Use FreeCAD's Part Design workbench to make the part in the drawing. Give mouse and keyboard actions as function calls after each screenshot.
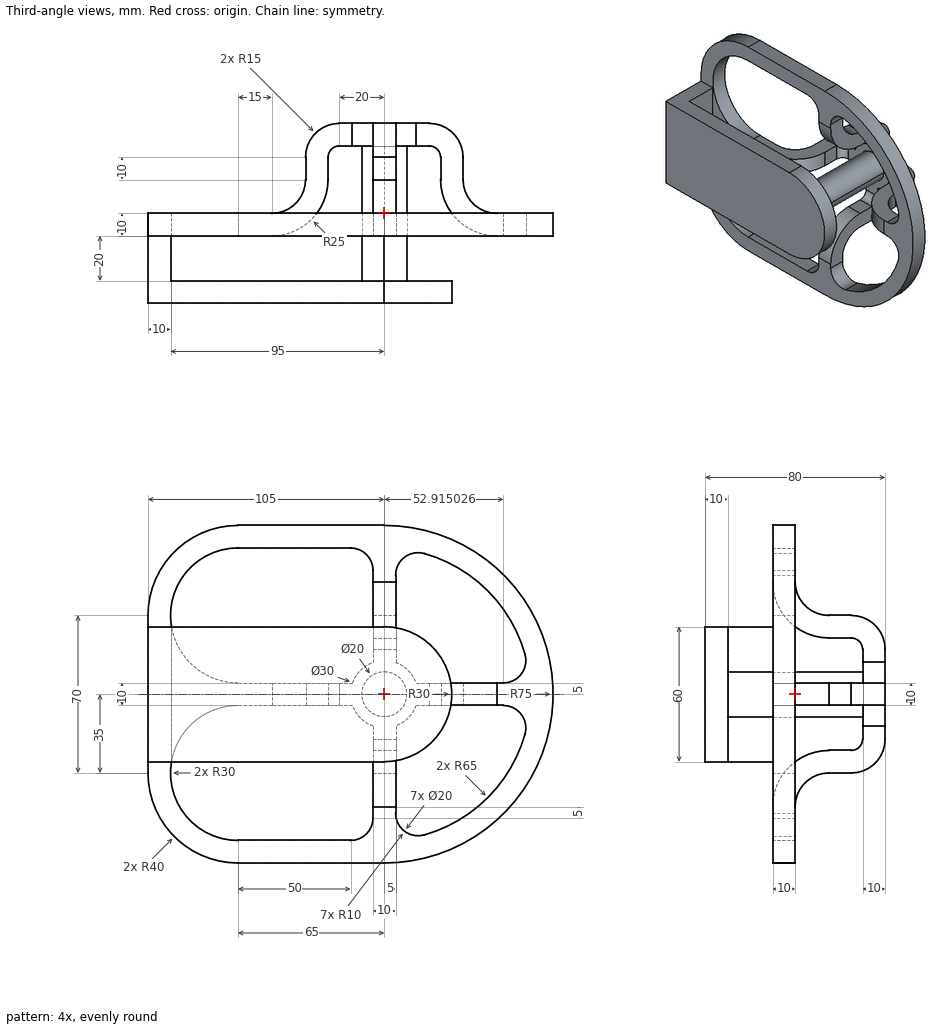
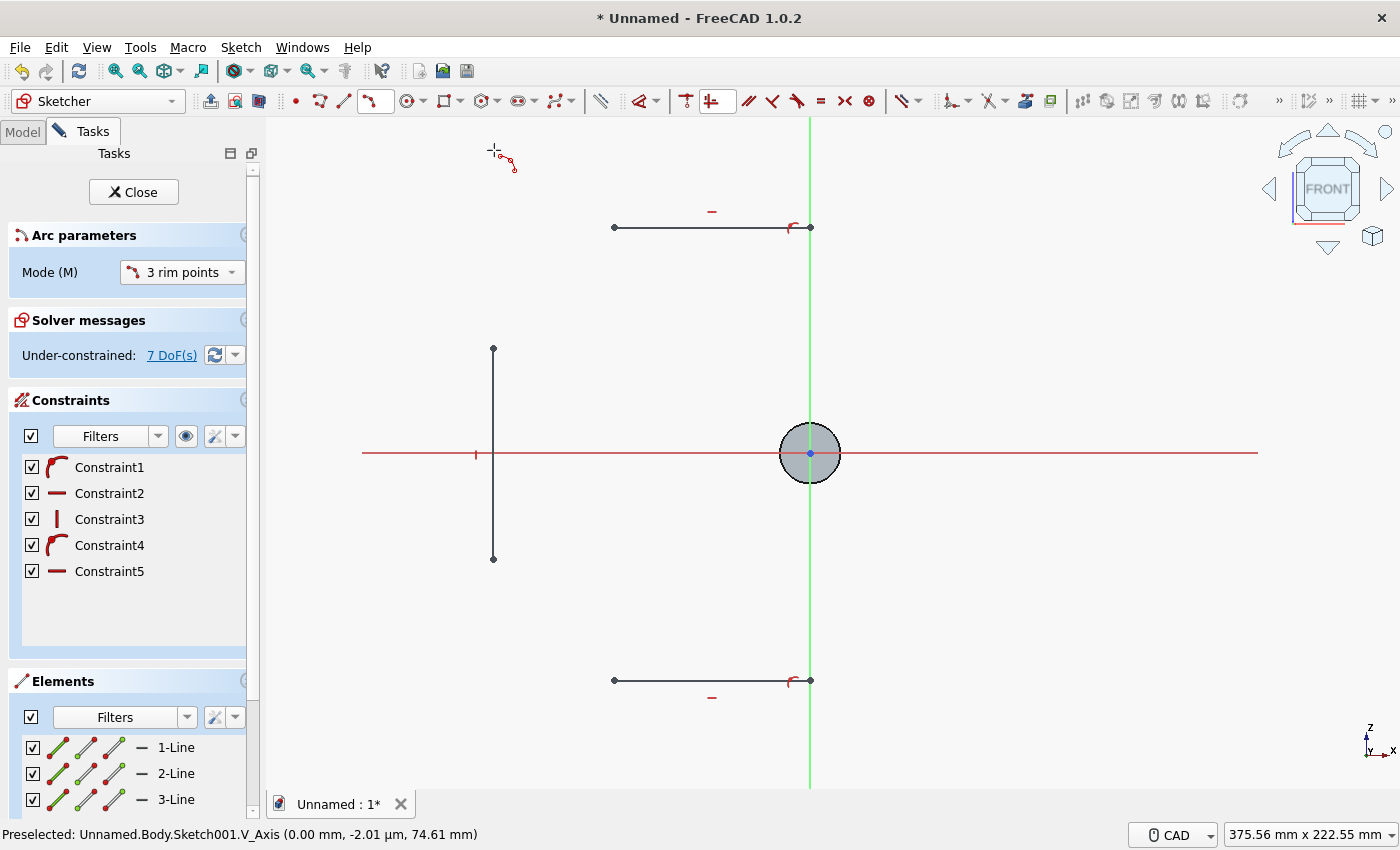
click(614, 681)
click(493, 560)
click(528, 644)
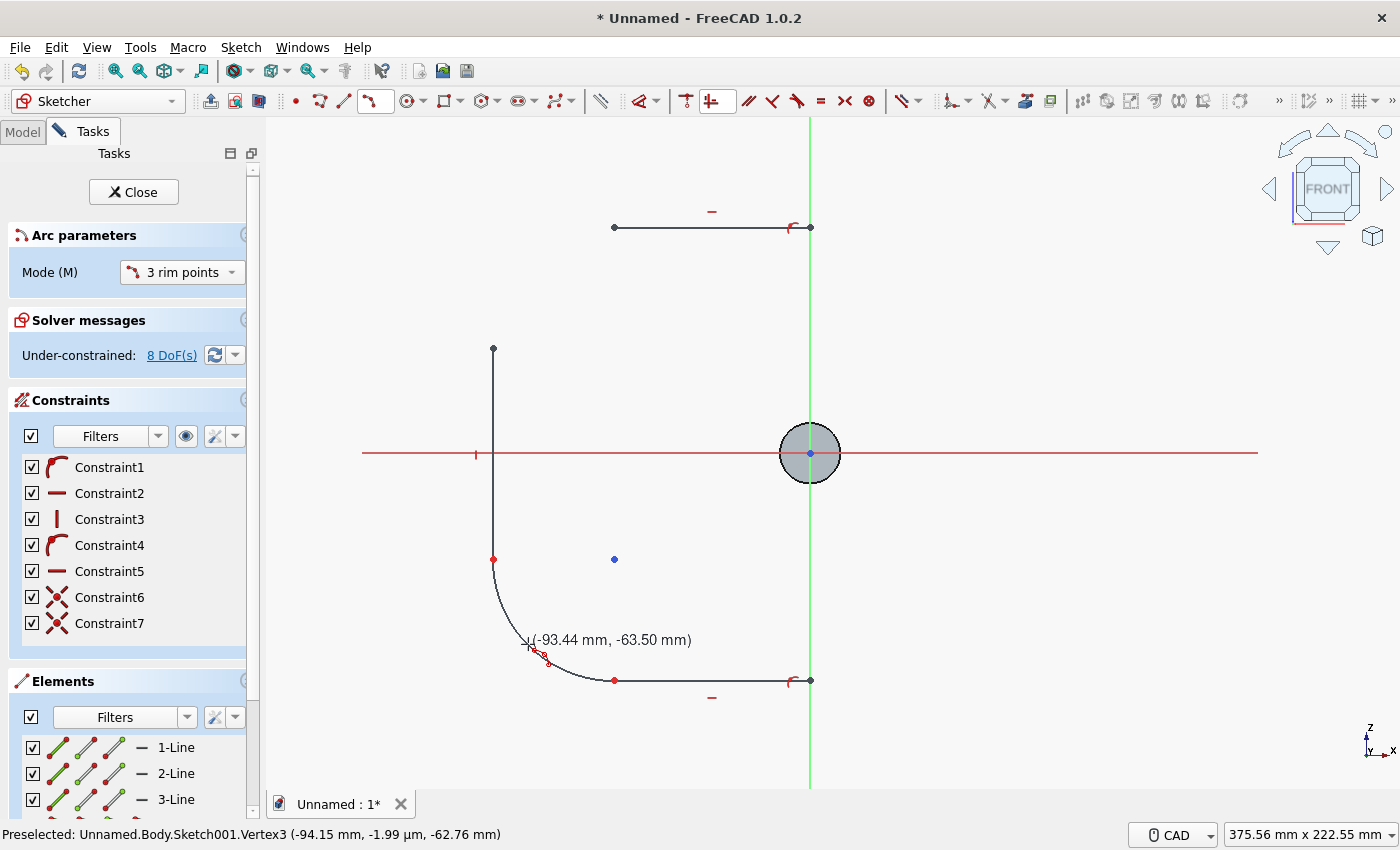
click(493, 349)
click(614, 228)
click(528, 262)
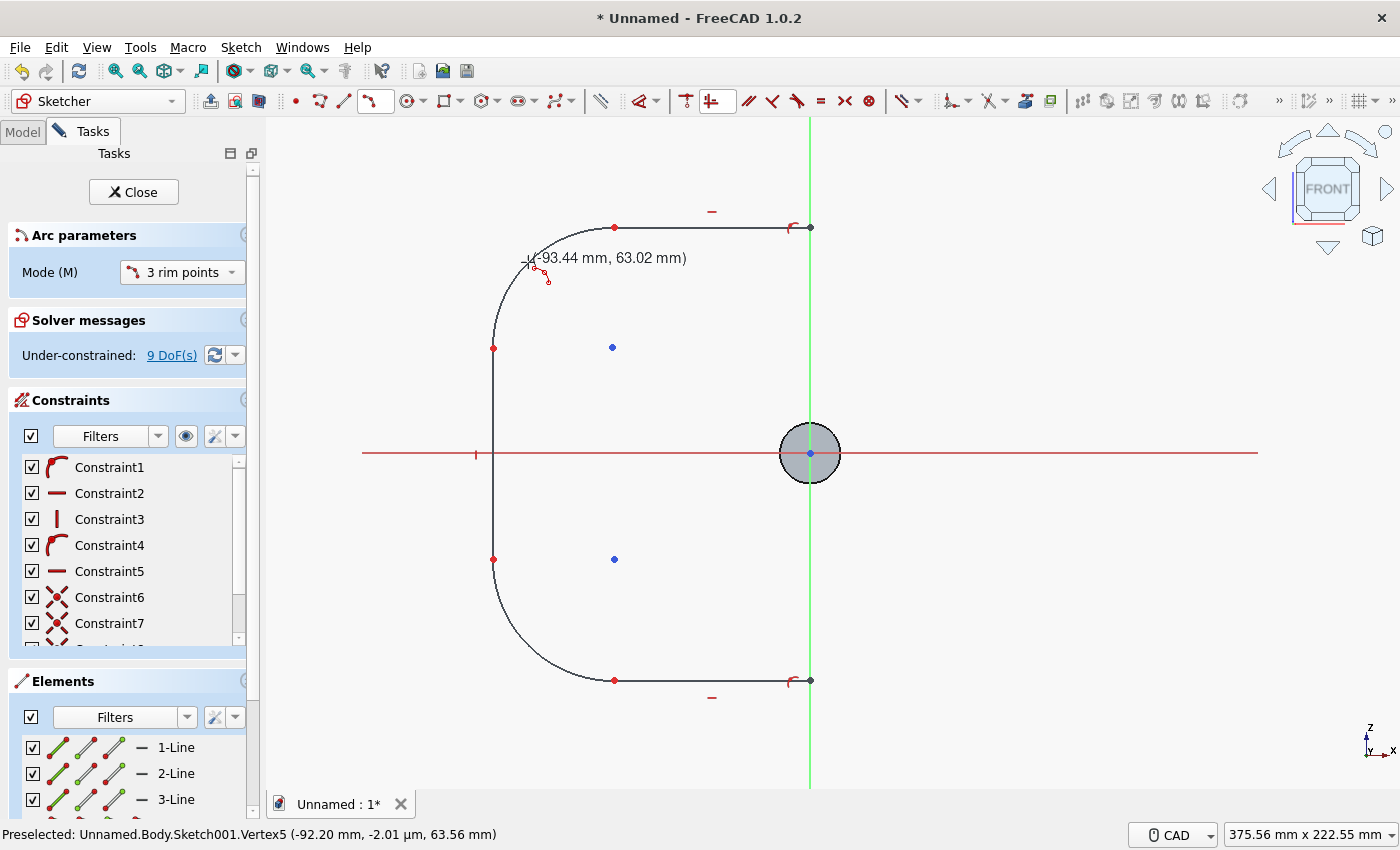
click(810, 228)
click(810, 681)
click(1026, 523)
key(Escape)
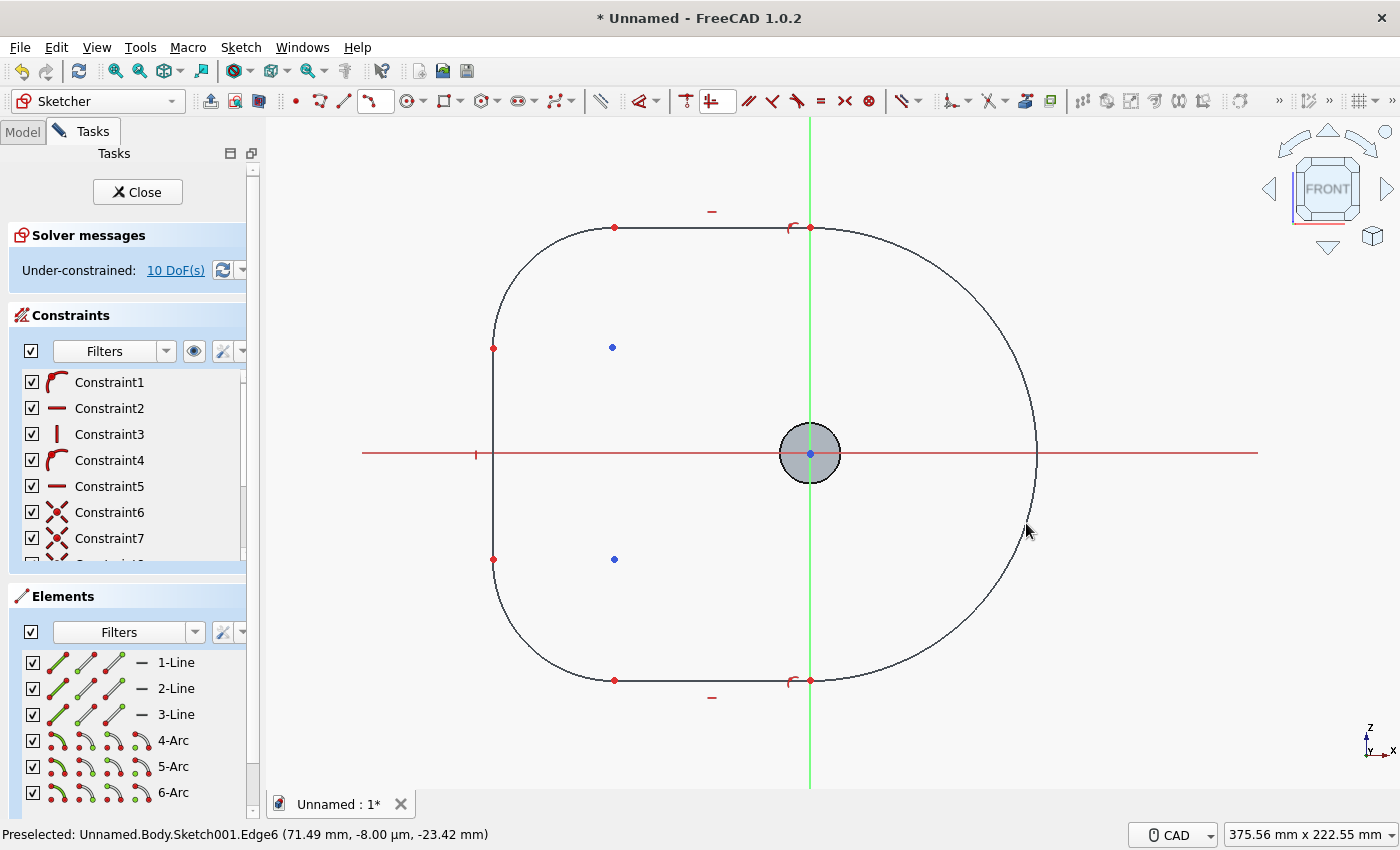
drag(800, 443, 820, 465)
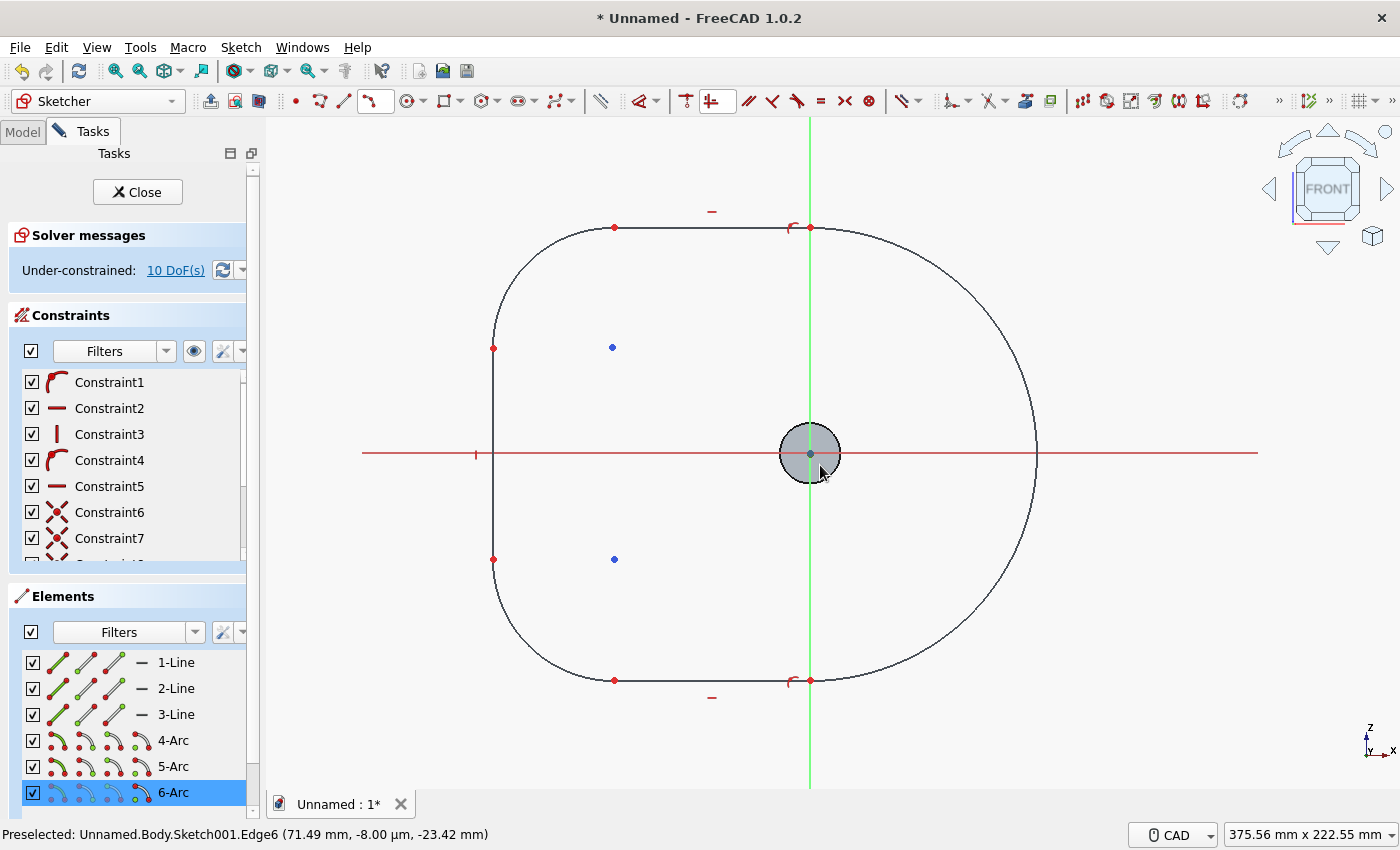
click(686, 102)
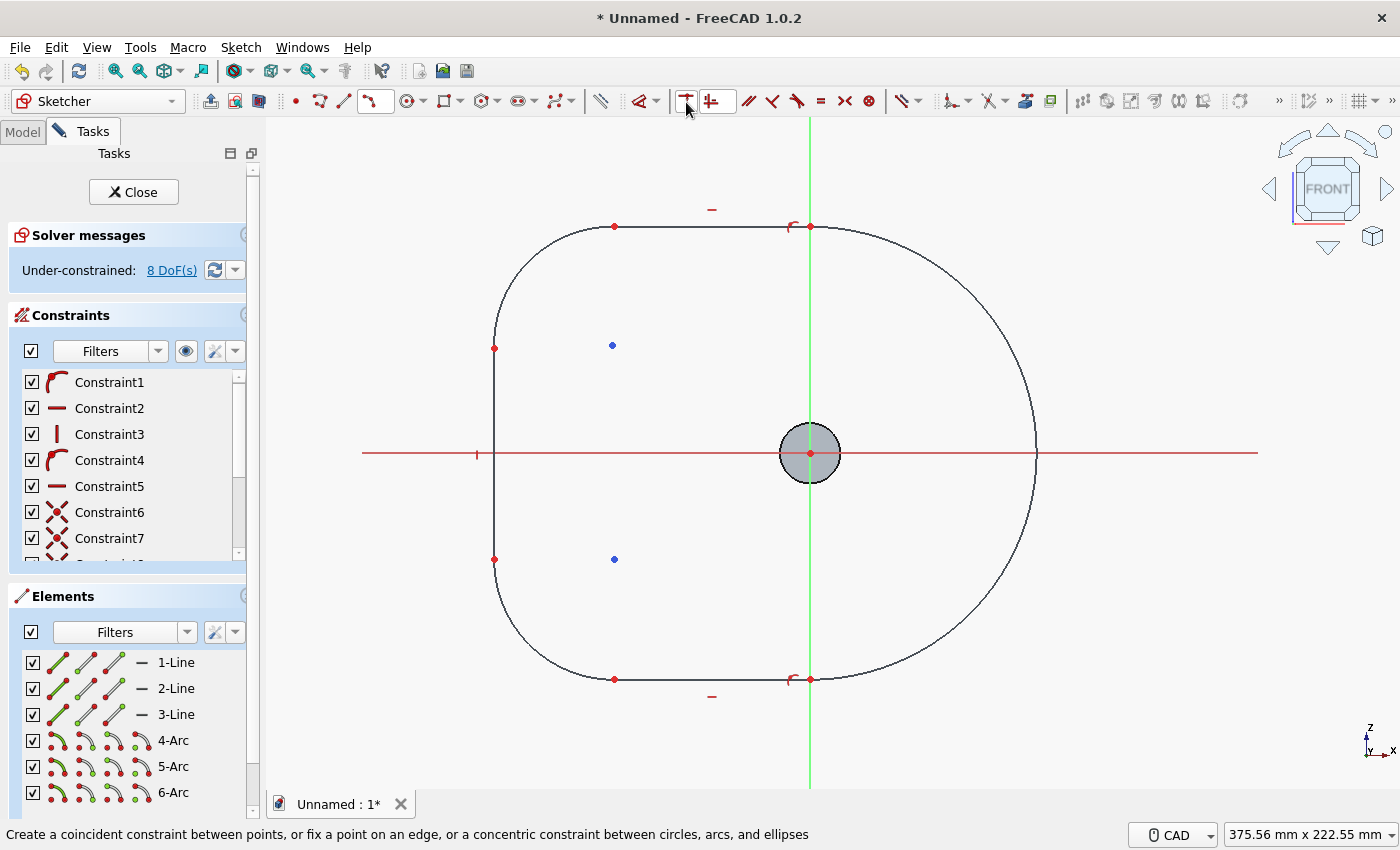
click(507, 614)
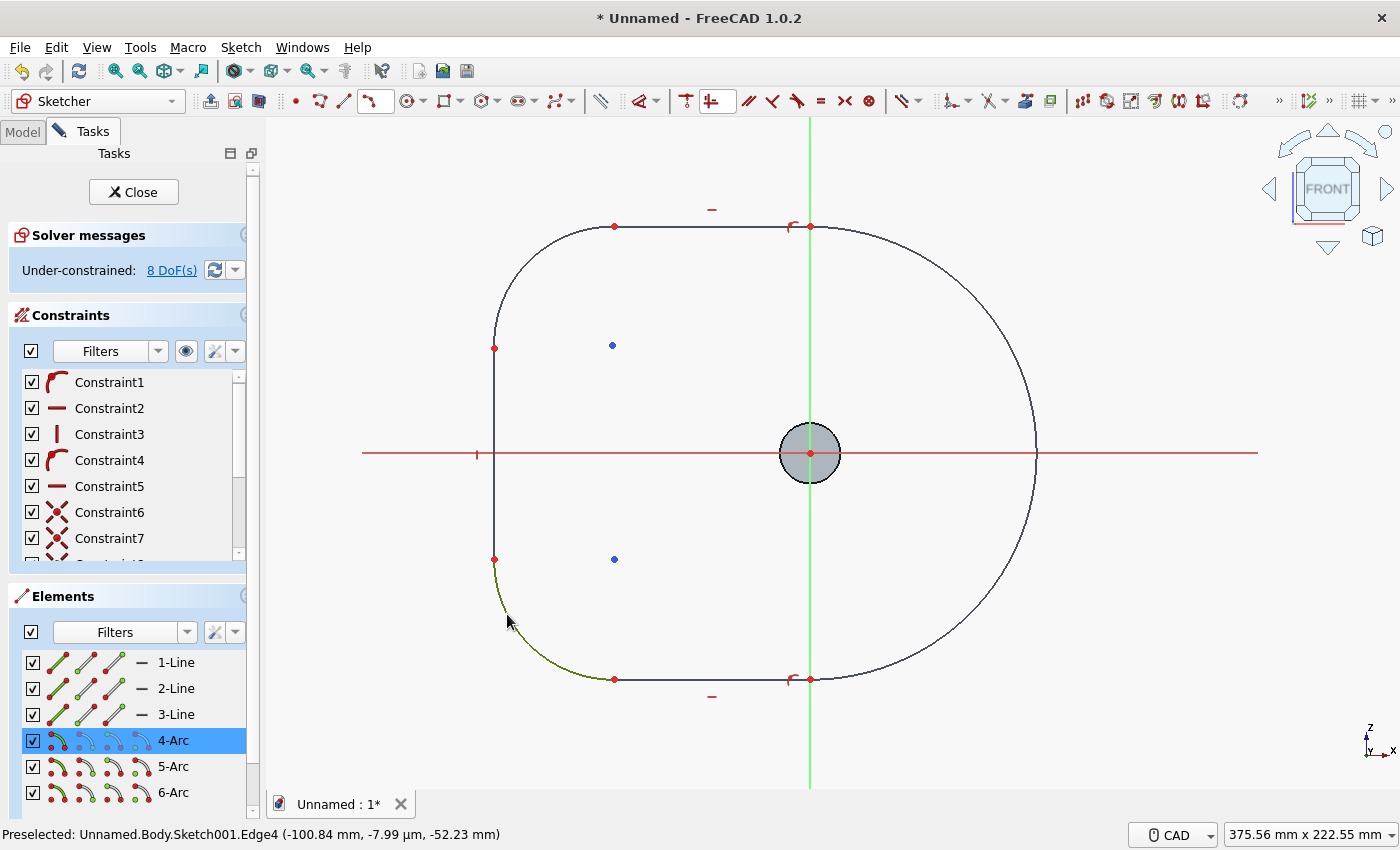
click(559, 240)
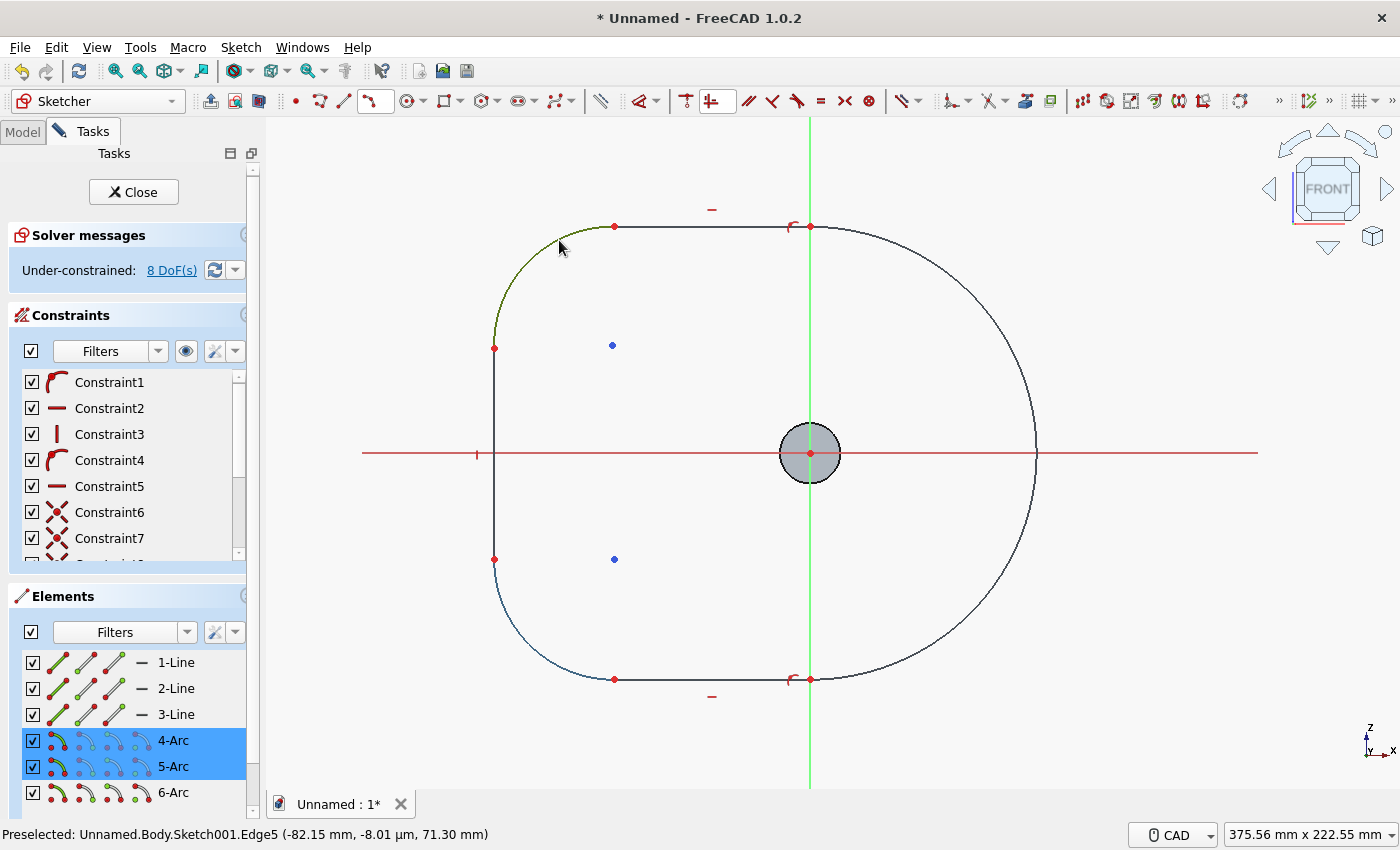
click(822, 102)